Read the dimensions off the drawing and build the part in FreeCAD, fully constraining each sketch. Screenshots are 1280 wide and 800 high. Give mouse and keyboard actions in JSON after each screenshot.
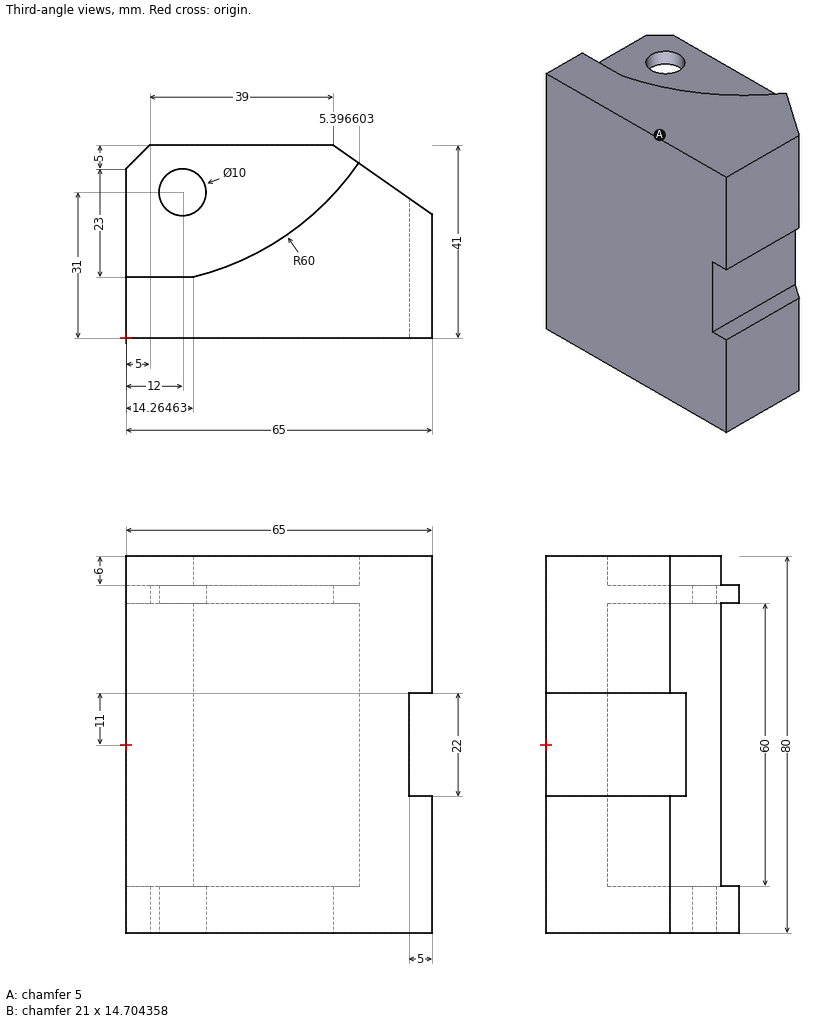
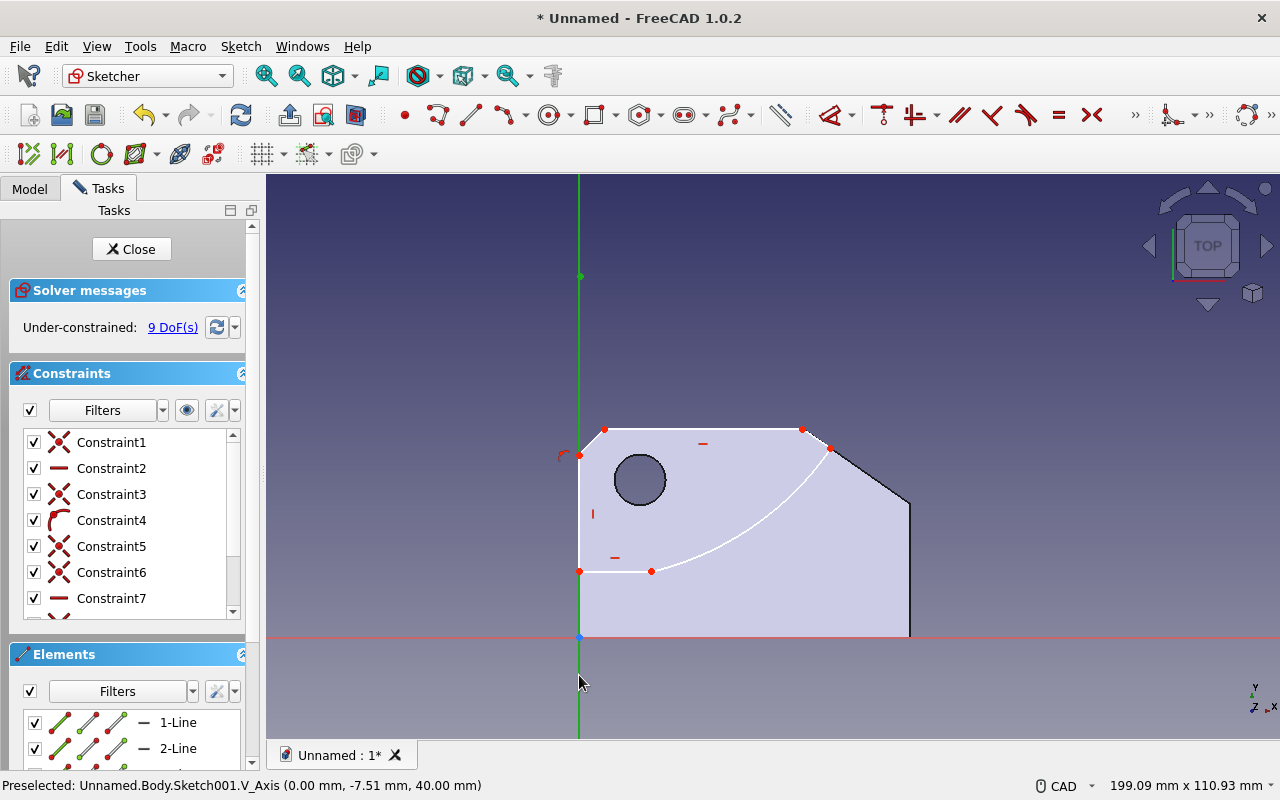
{"action": "left_click", "coordinate": [882, 116]}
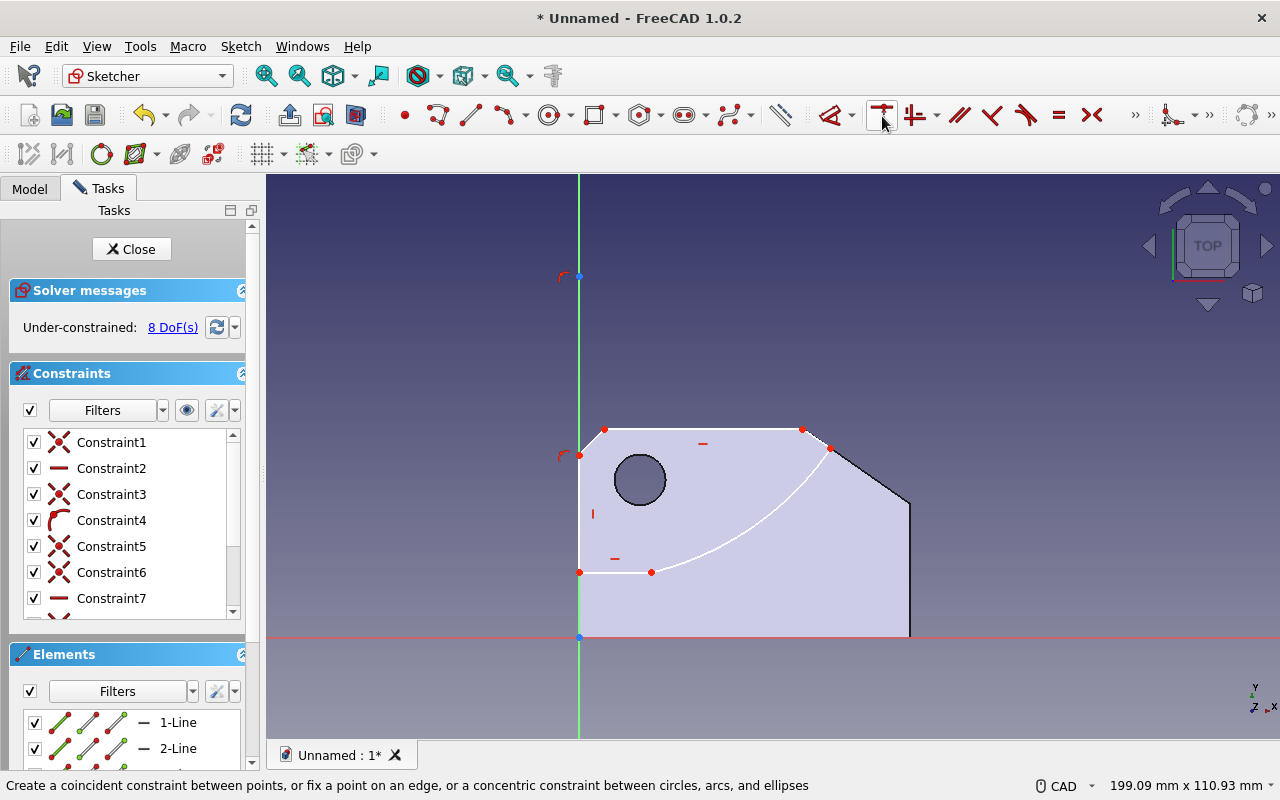
{"action": "left_click", "coordinate": [830, 116]}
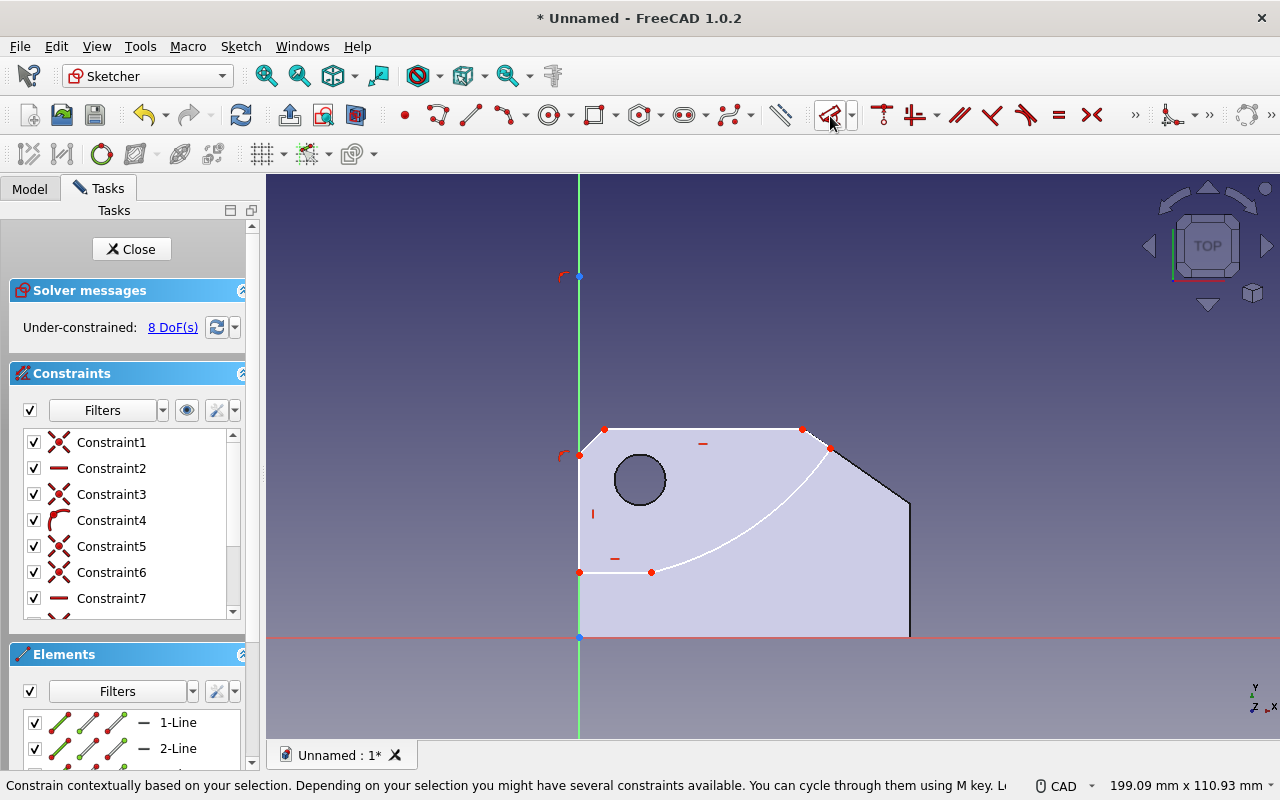
{"action": "left_click", "coordinate": [714, 550]}
{"action": "left_click", "coordinate": [728, 579]}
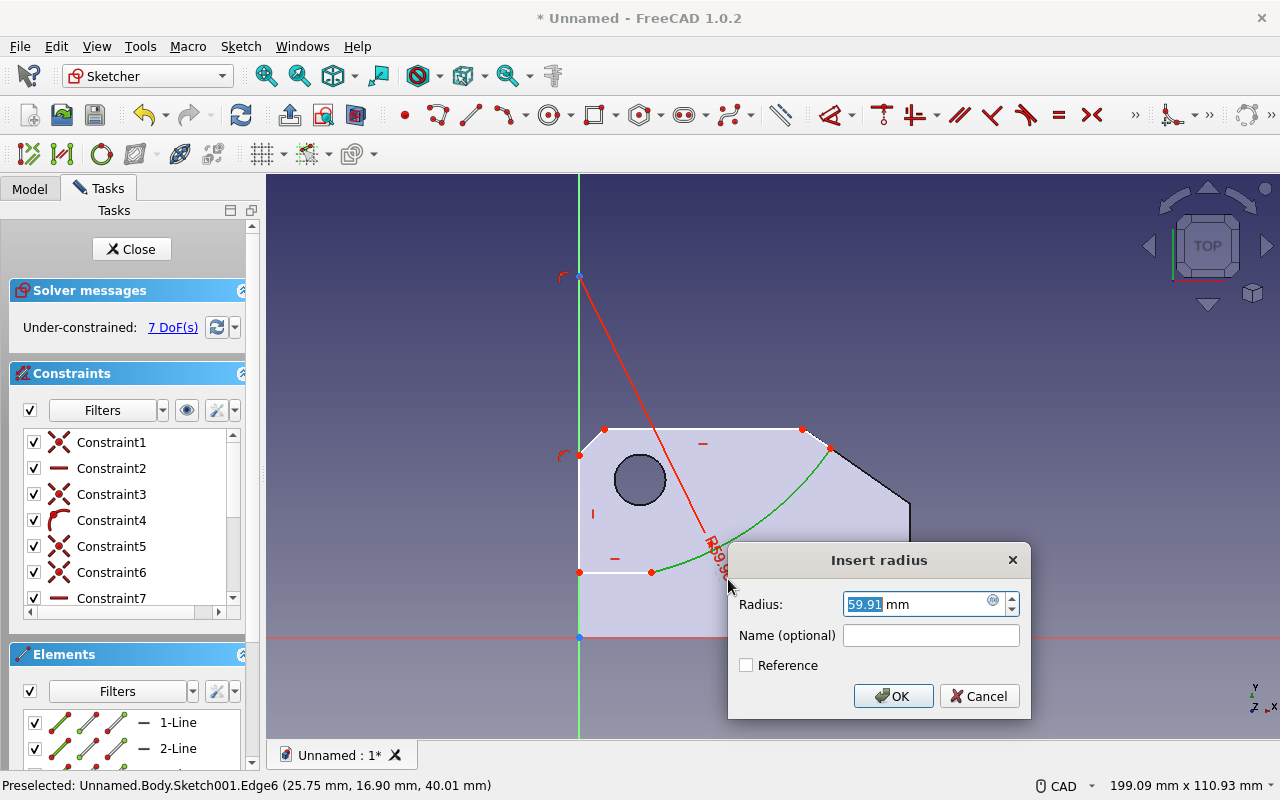
{"action": "type", "text": "60"}
{"action": "key", "text": "Return"}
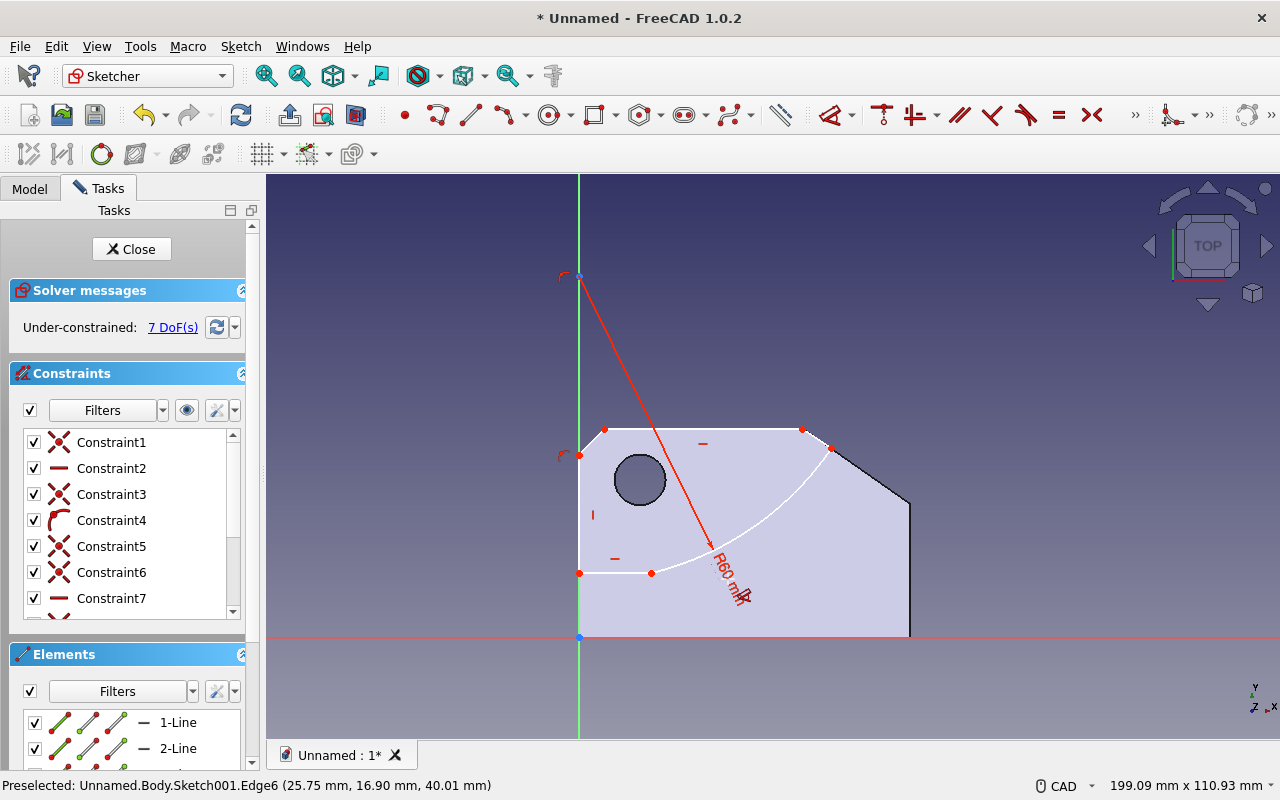
{"action": "left_click", "coordinate": [743, 429]}
{"action": "left_click", "coordinate": [704, 395]}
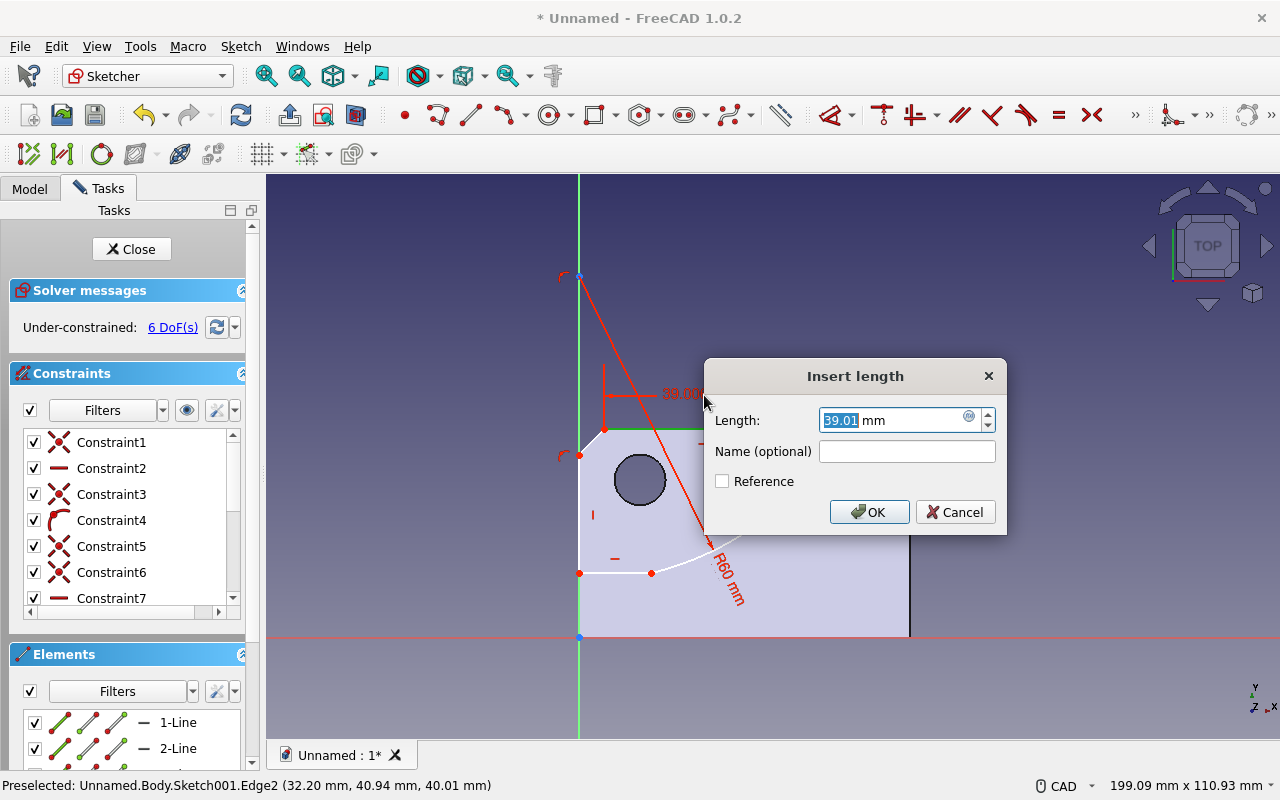
{"action": "type", "text": "39"}
{"action": "key", "text": "Return"}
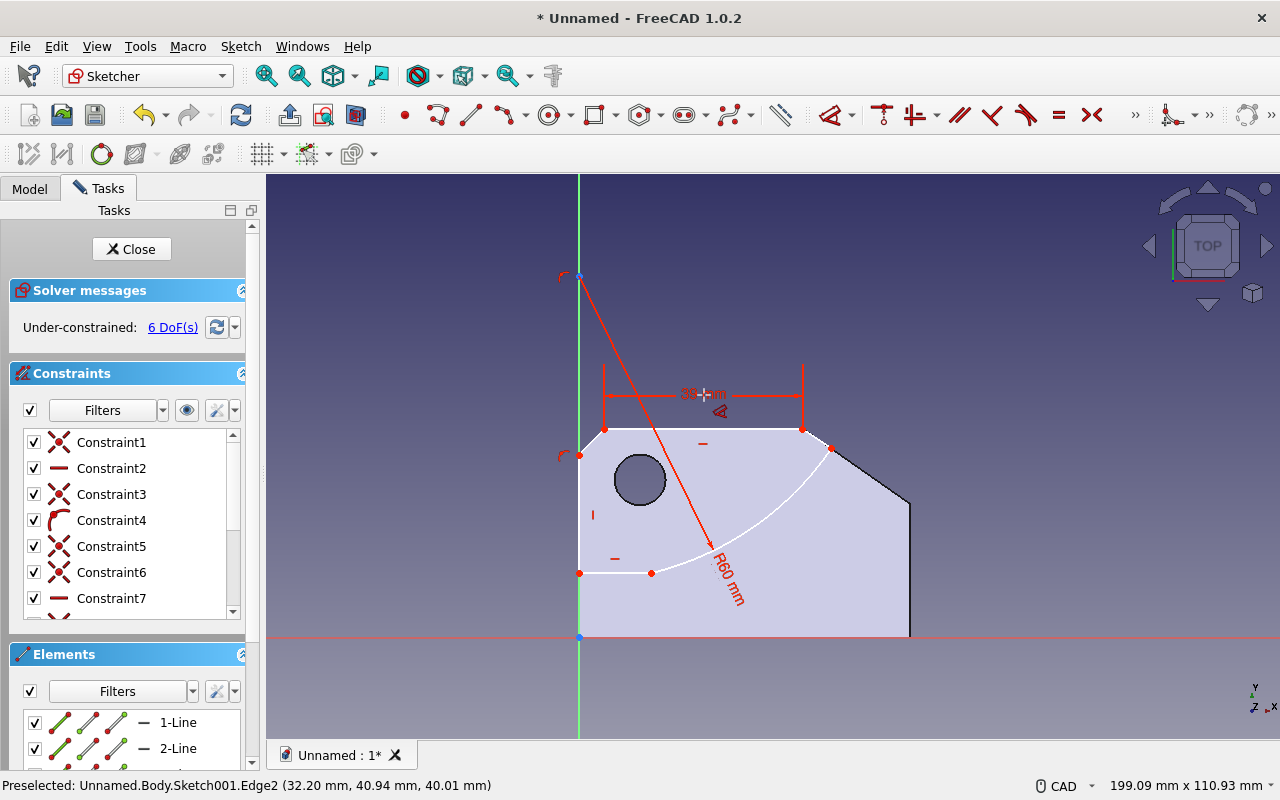
{"action": "left_click", "coordinate": [579, 490]}
{"action": "left_click", "coordinate": [545, 514]}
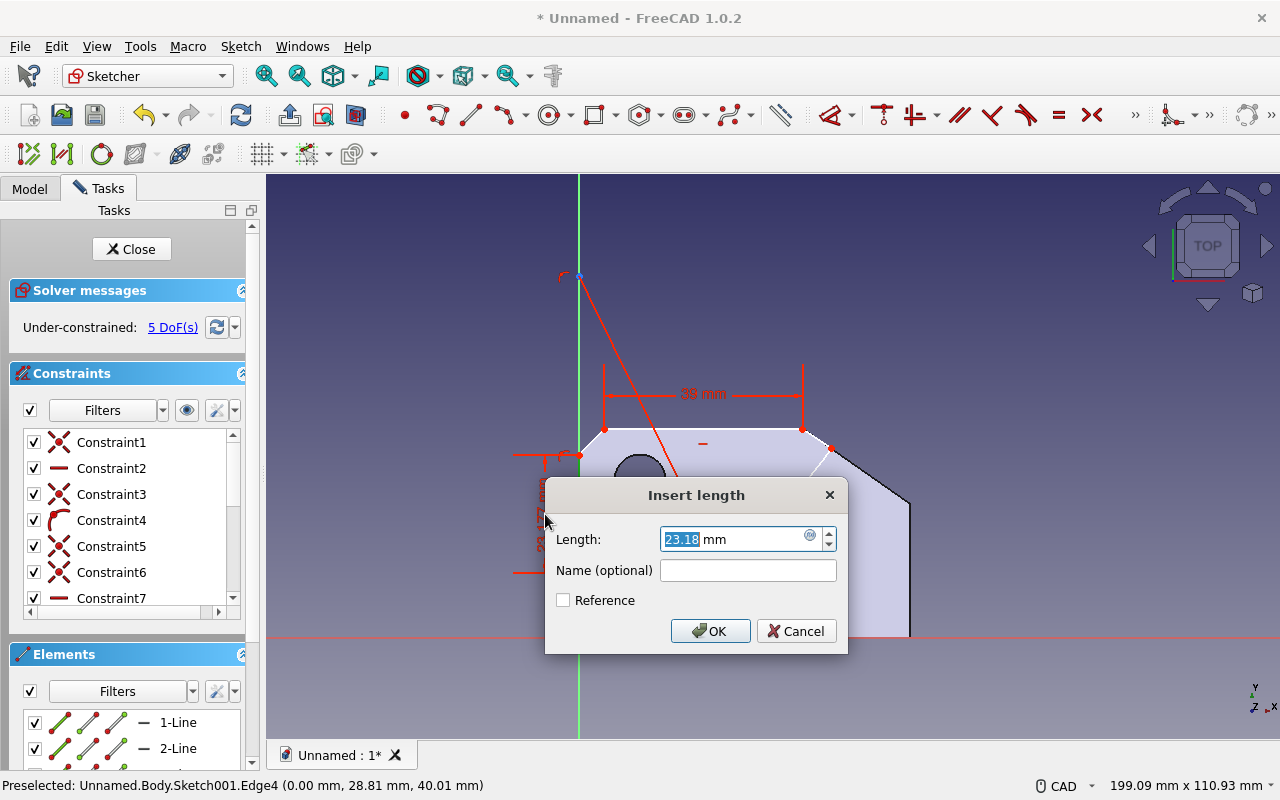
{"action": "type", "text": "23"}
{"action": "key", "text": "Return"}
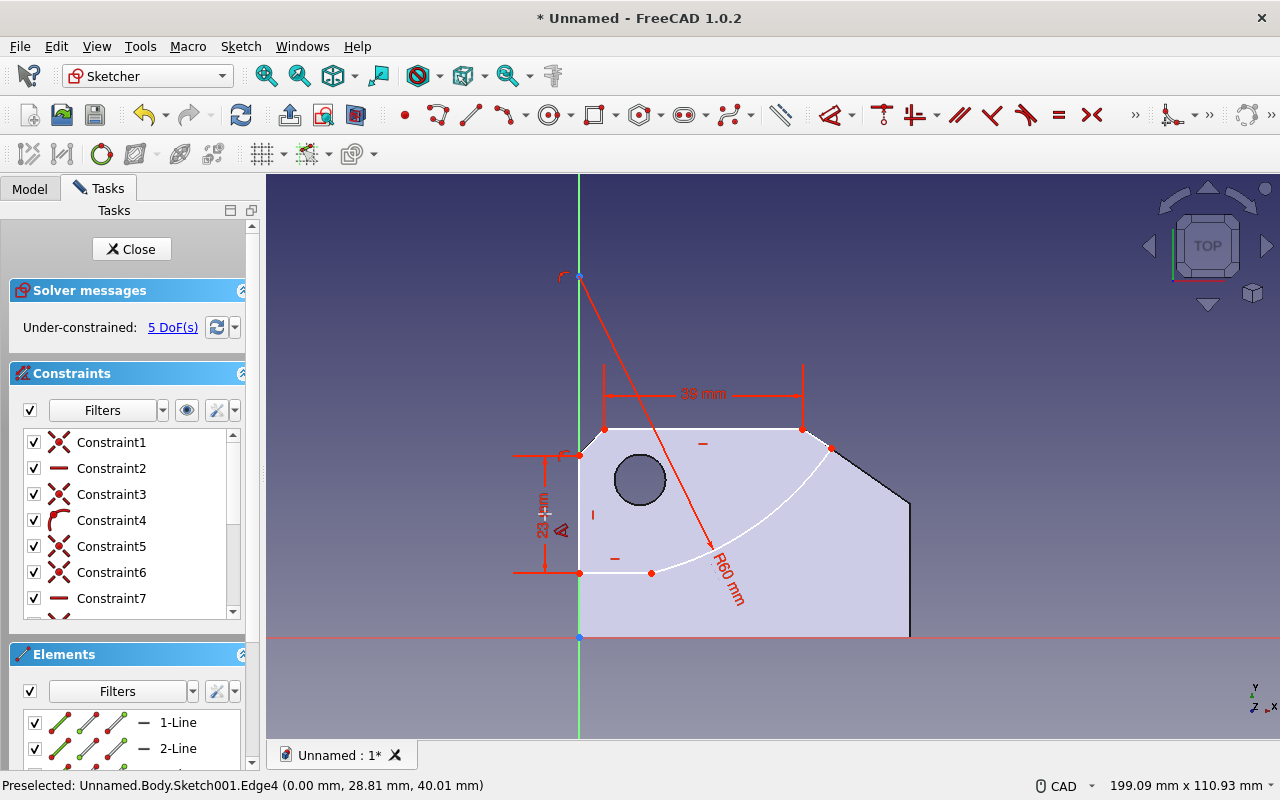
{"action": "scroll", "coordinate": [604, 429], "scroll_direction": "up", "scroll_amount": 3}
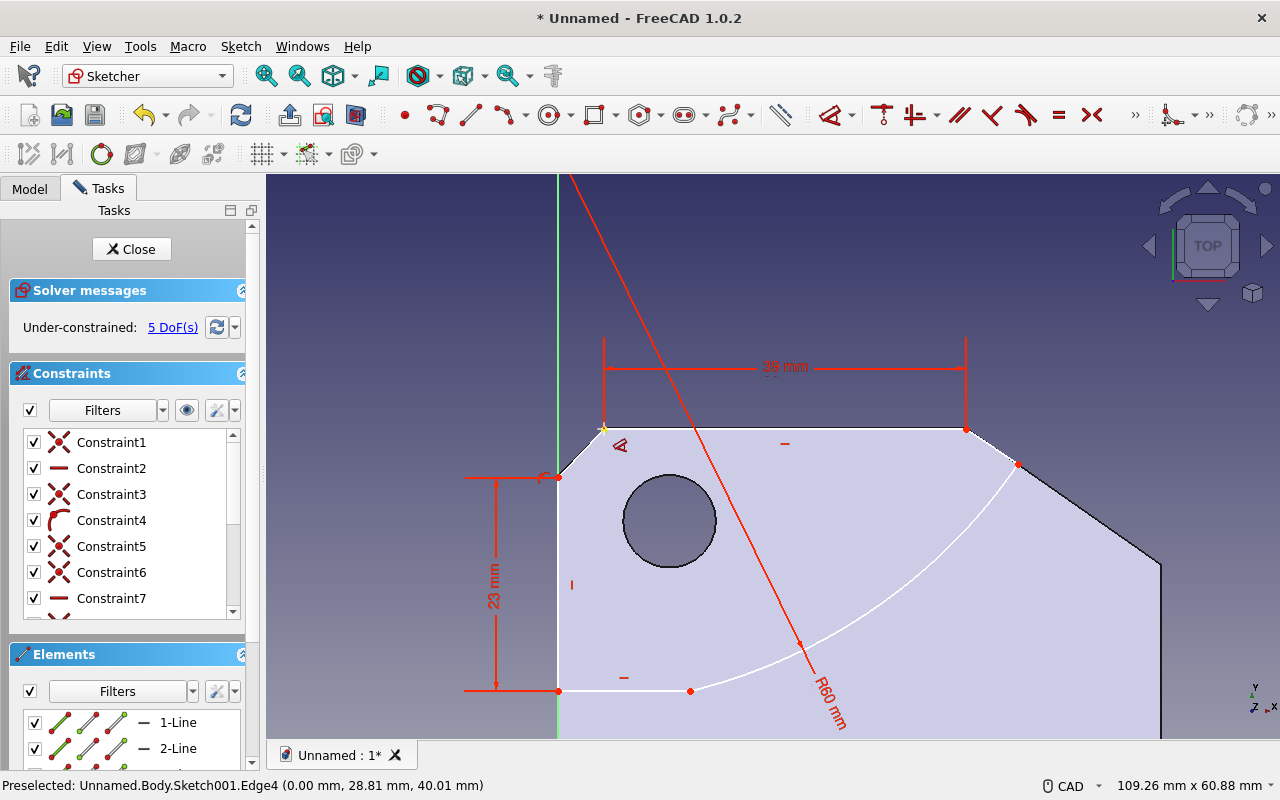
{"action": "left_click", "coordinate": [604, 429]}
{"action": "left_click", "coordinate": [581, 395]}